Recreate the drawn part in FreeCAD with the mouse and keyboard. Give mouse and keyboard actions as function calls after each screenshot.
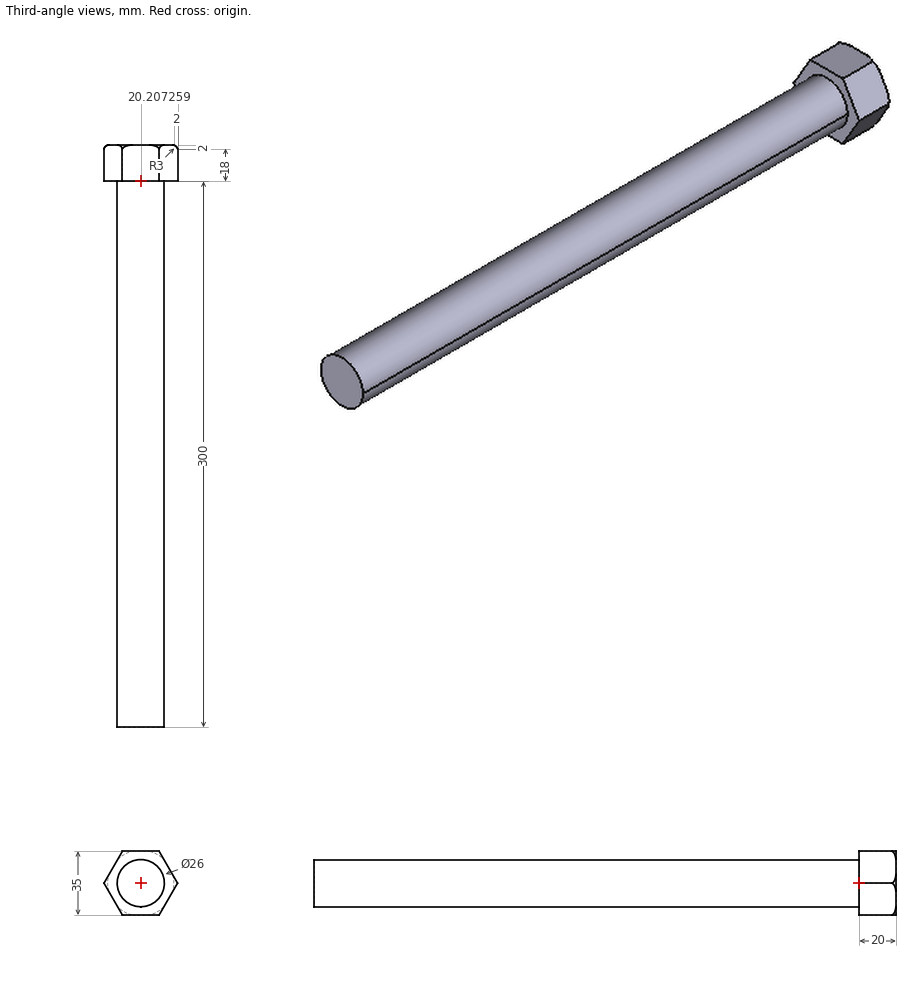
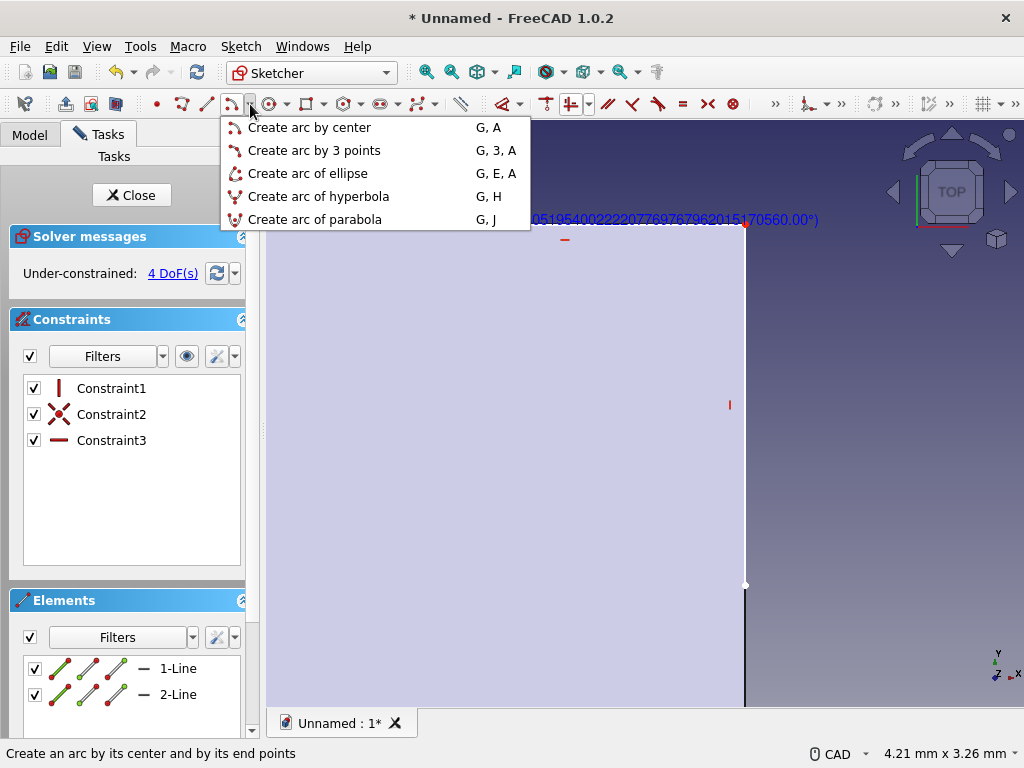
click(376, 150)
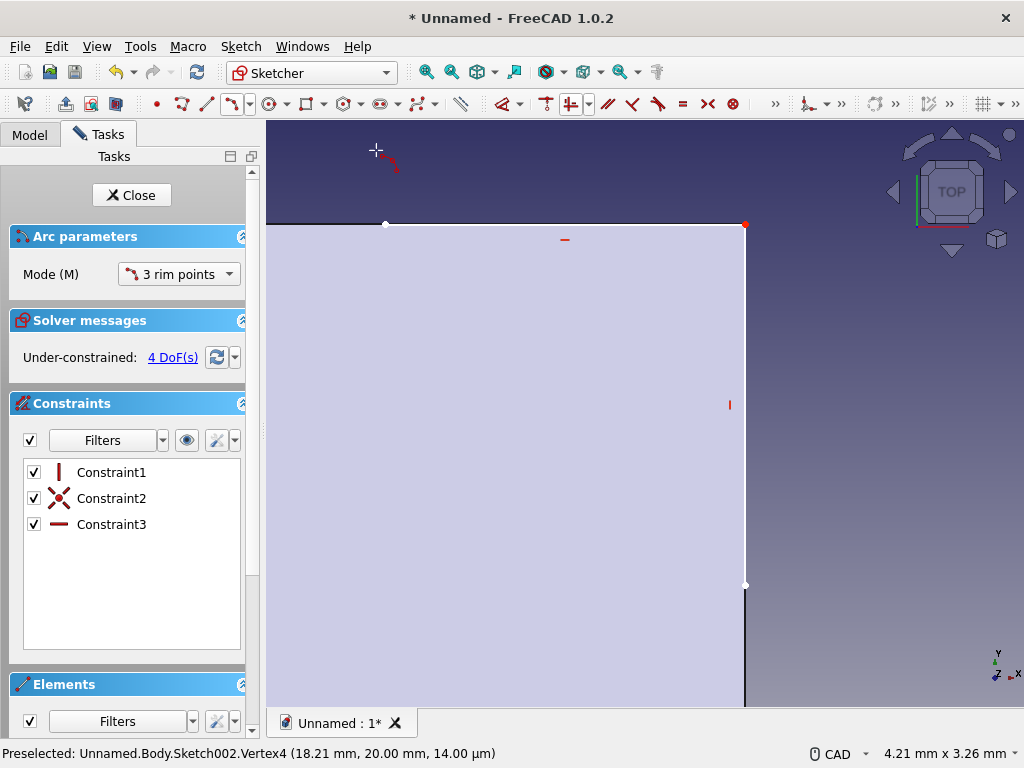
click(385, 225)
click(745, 585)
click(610, 359)
key(Escape)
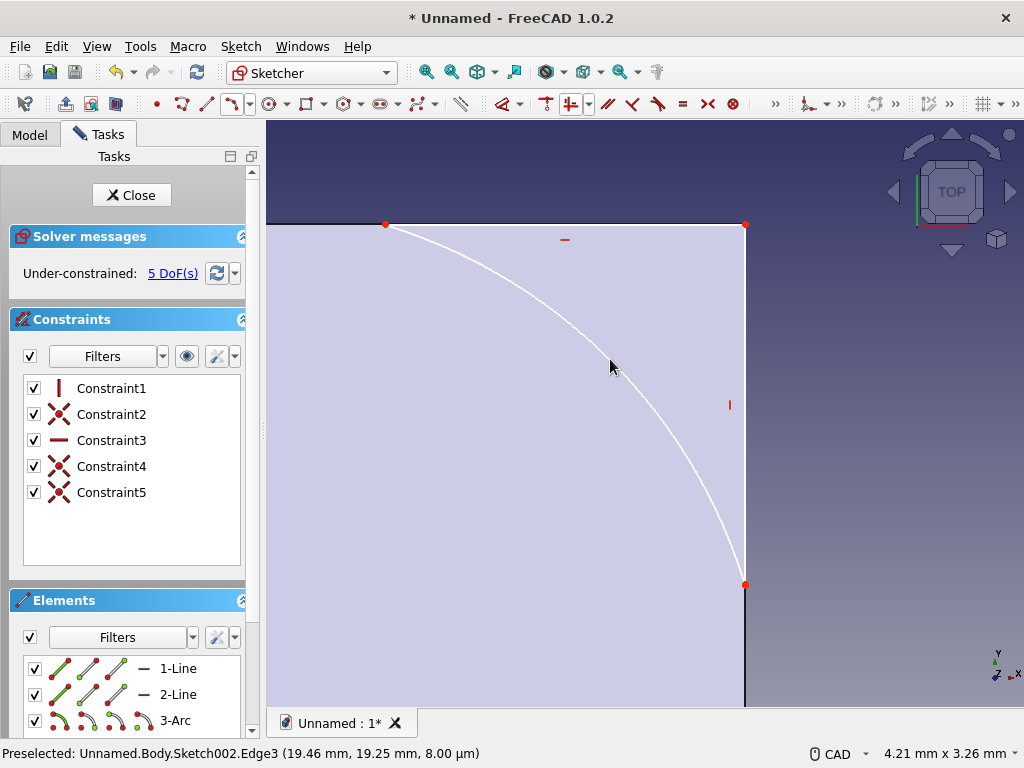
click(502, 104)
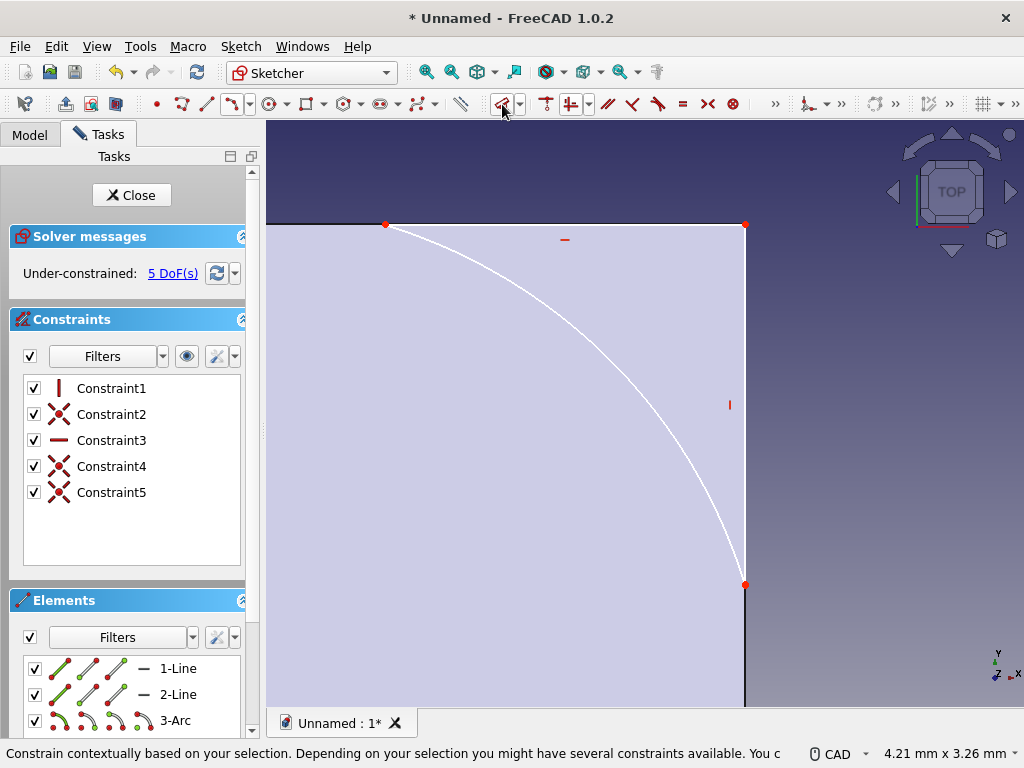
click(677, 442)
click(704, 424)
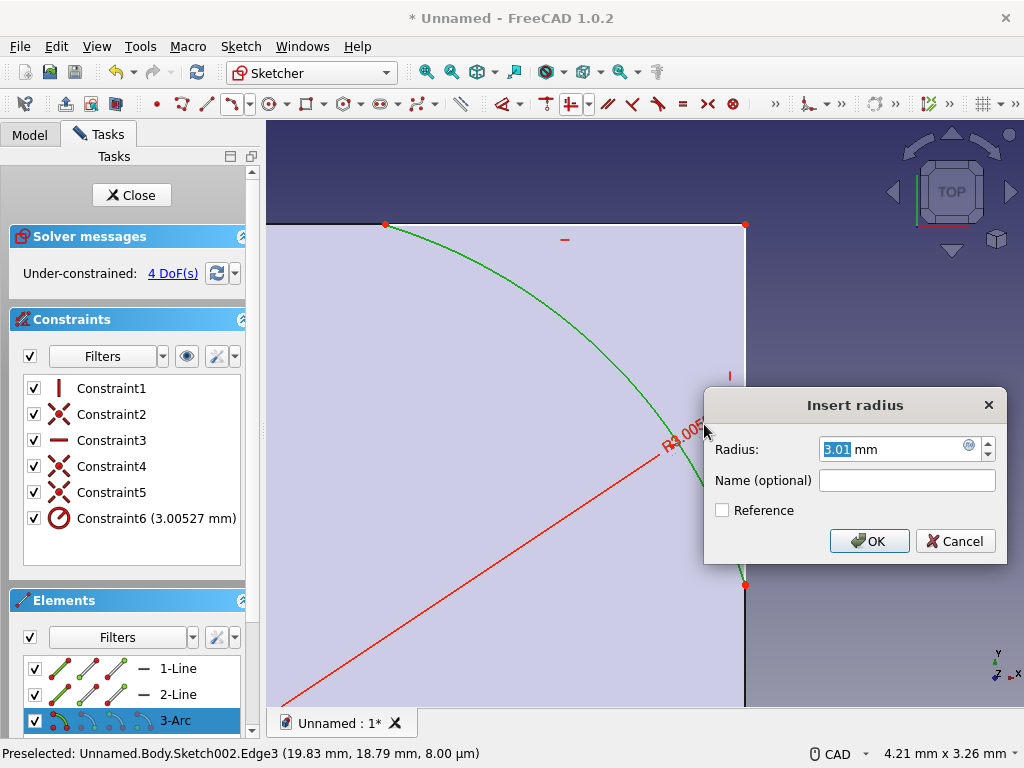
text(3)
key(Return)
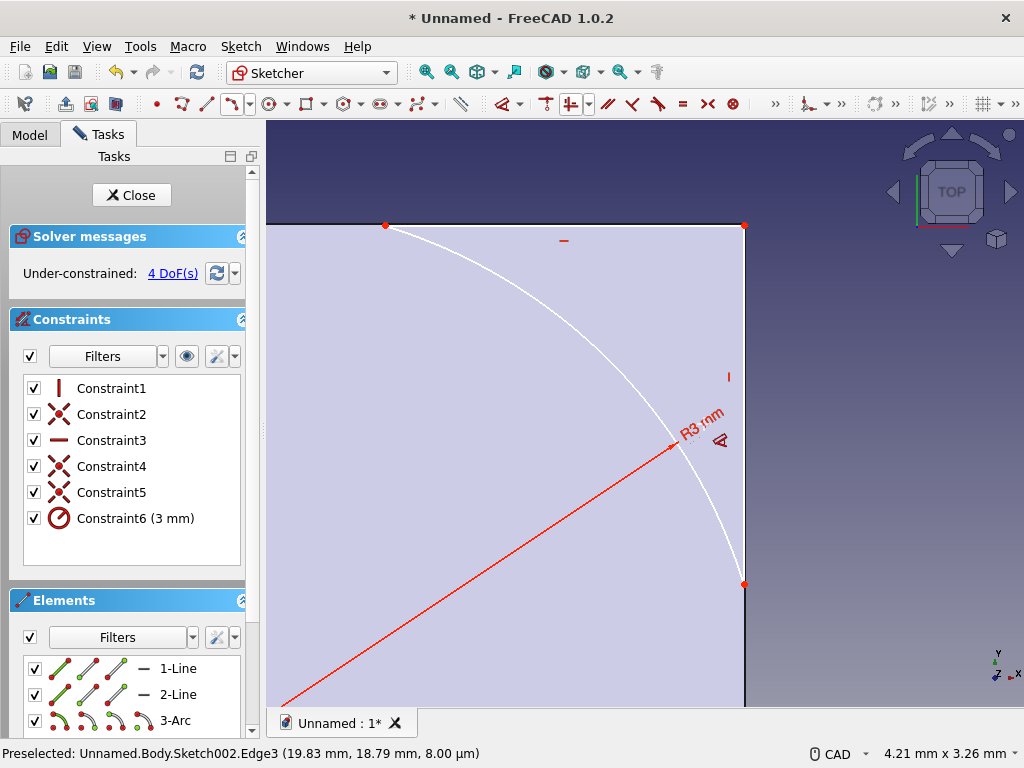
click(744, 477)
click(778, 405)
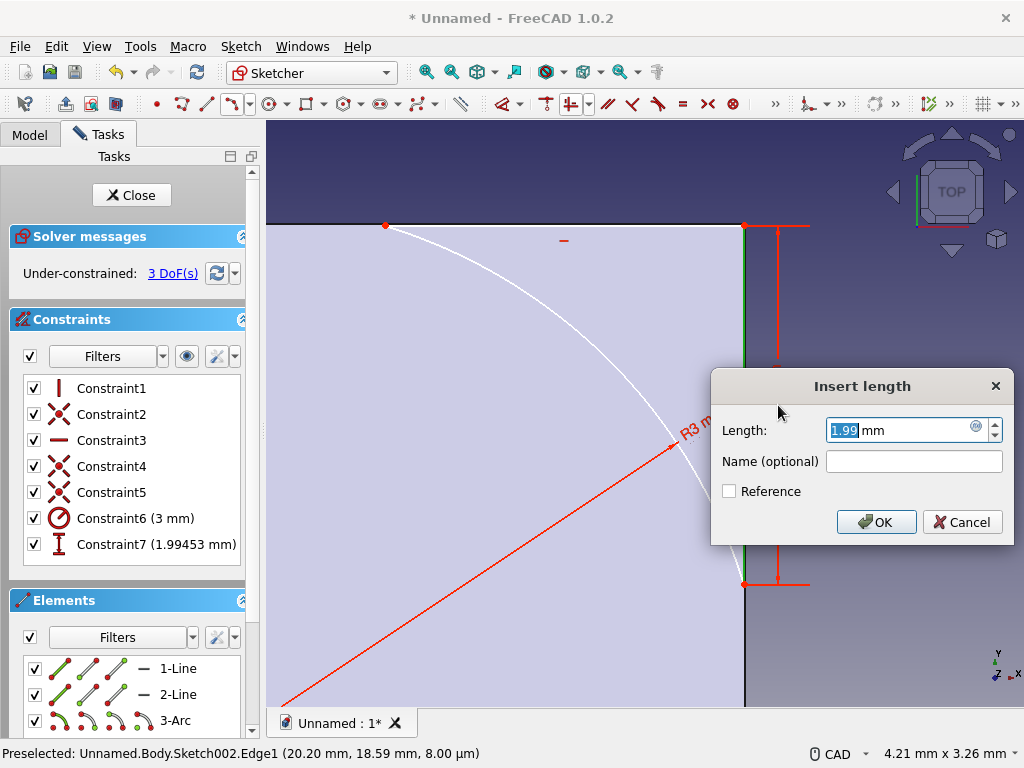
text(2)
key(Return)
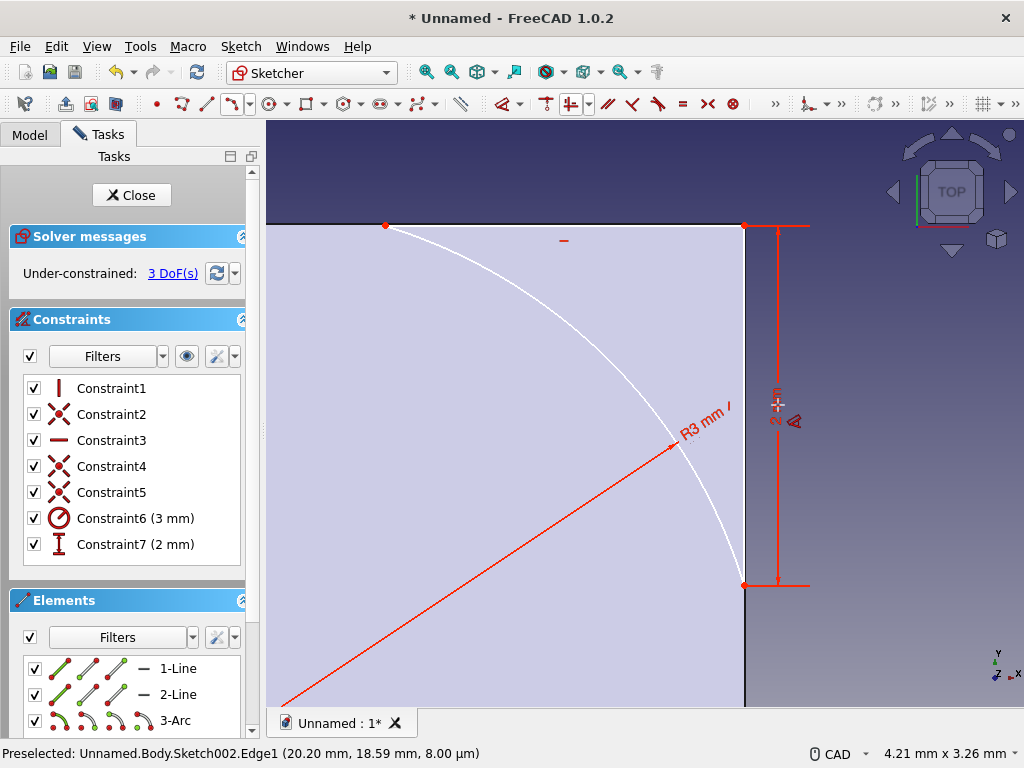
click(637, 226)
click(565, 192)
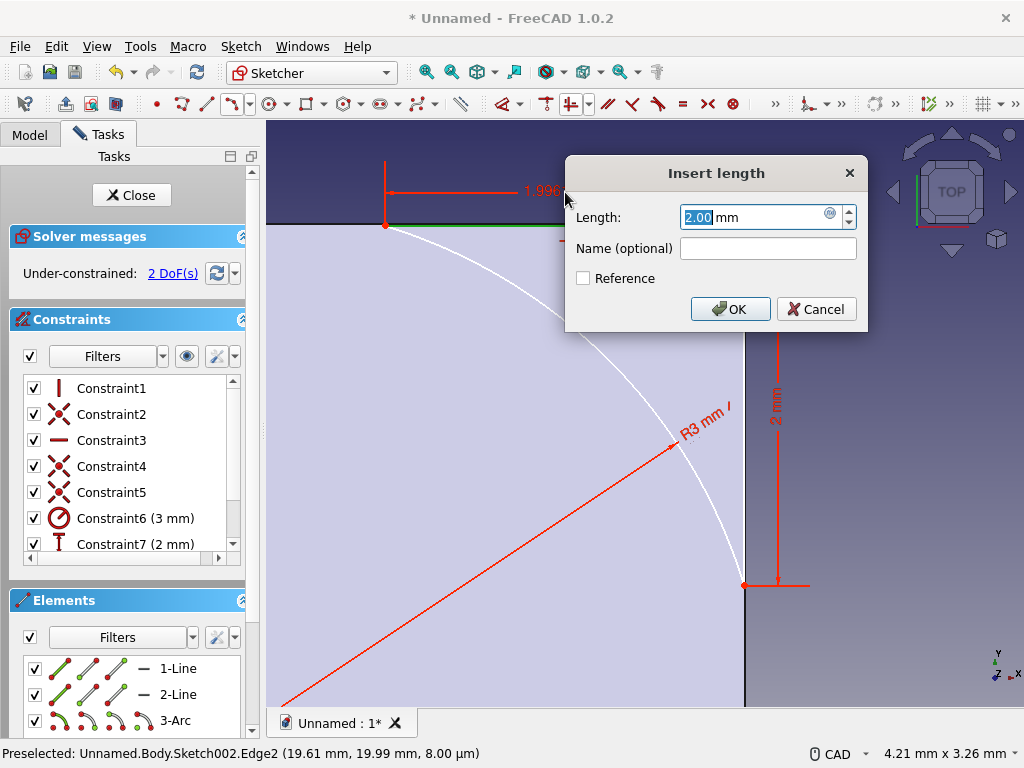
text(2)
key(Return)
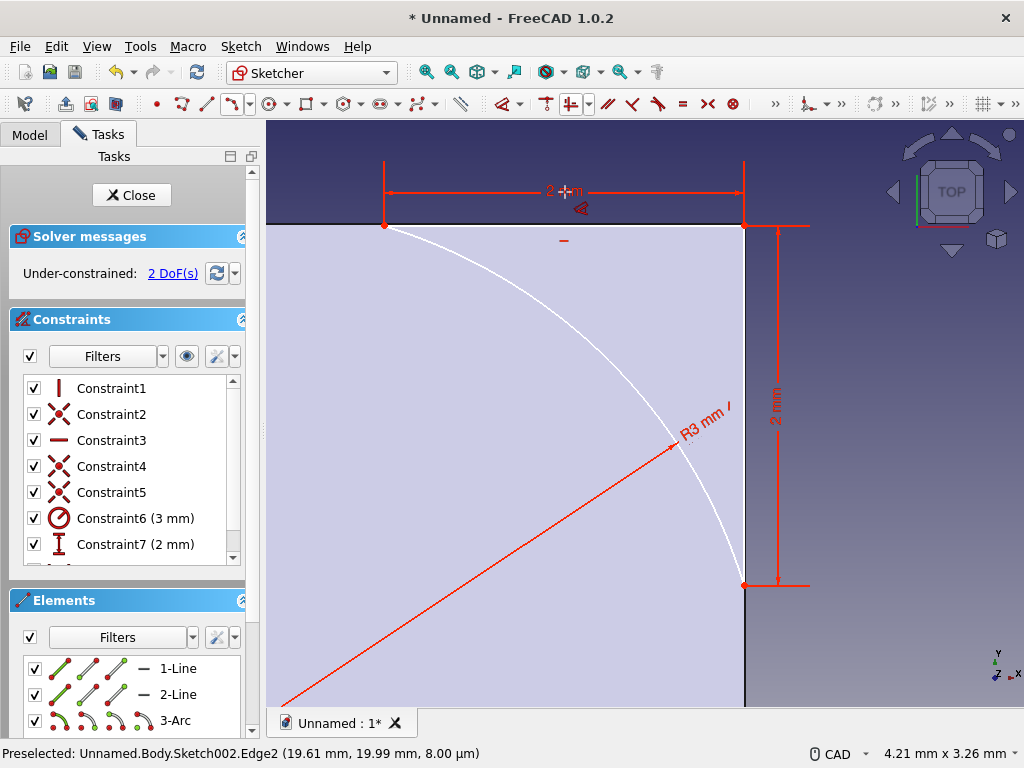
click(744, 586)
click(778, 632)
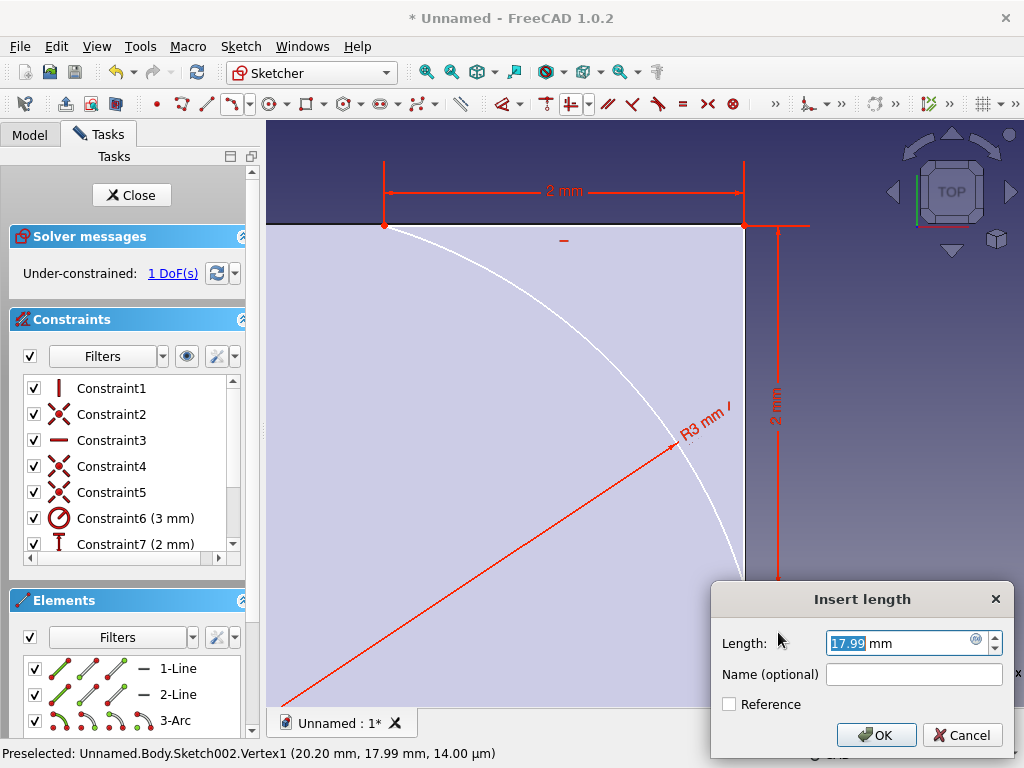
text(18)
key(Return)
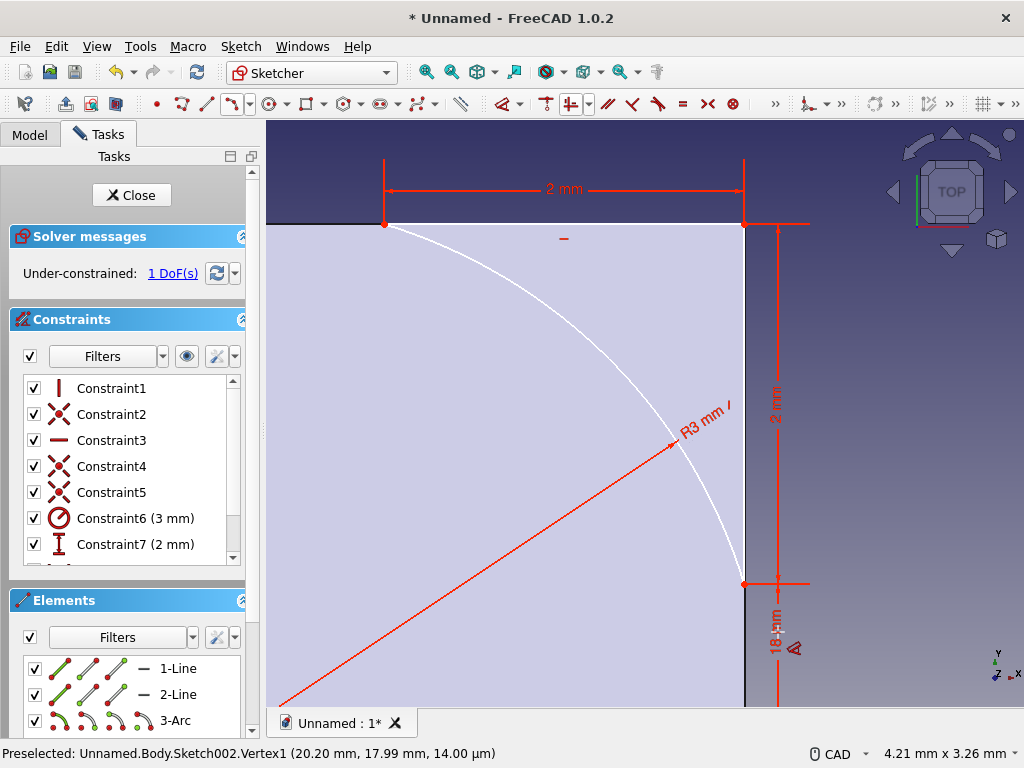
click(744, 584)
click(519, 550)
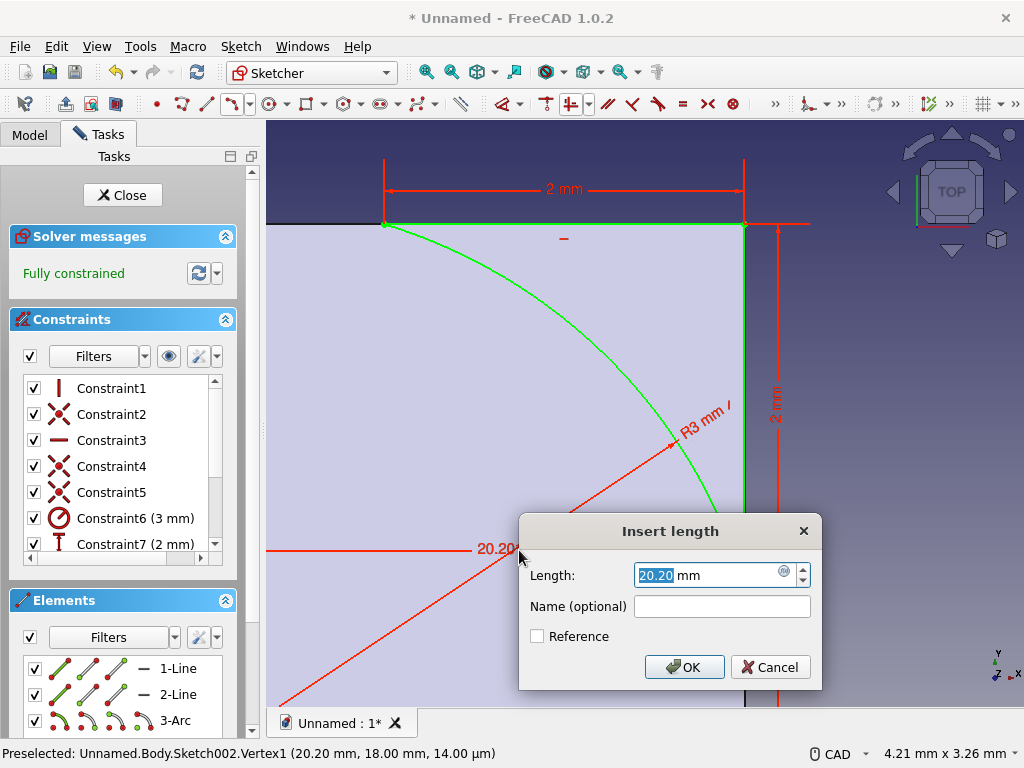
text(20.207259)
key(Return)
key(Escape)